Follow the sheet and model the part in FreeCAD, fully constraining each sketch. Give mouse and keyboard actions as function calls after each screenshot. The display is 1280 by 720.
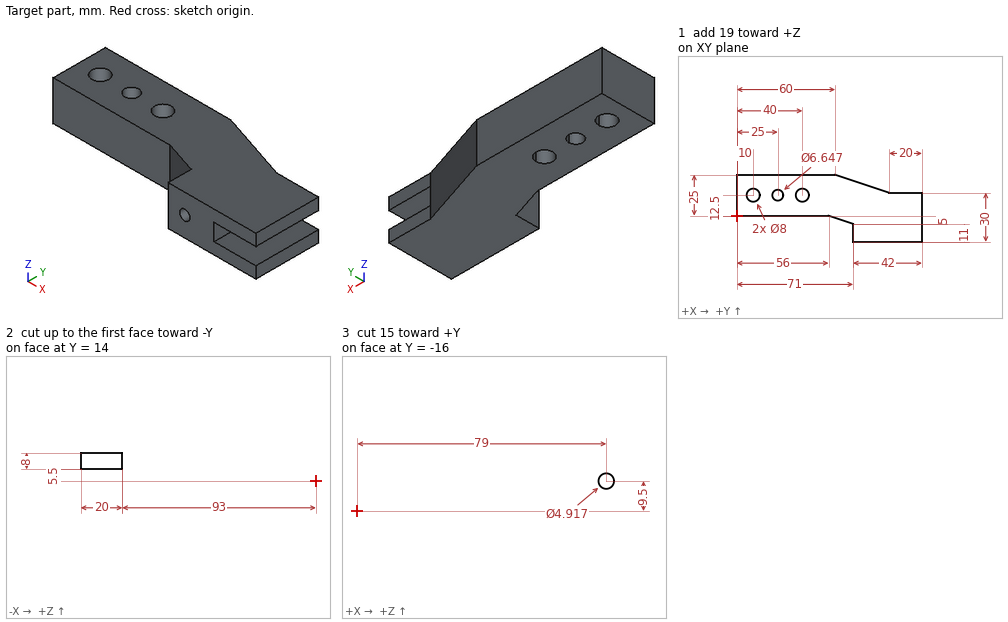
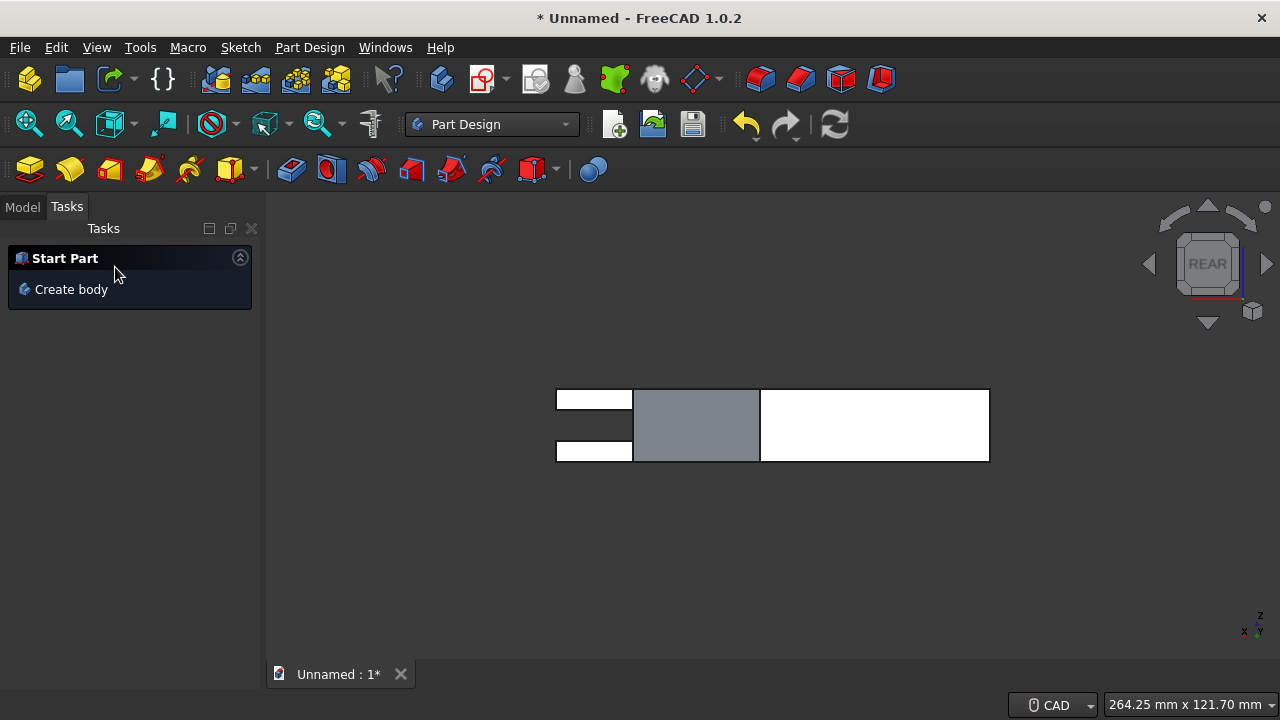
key(0)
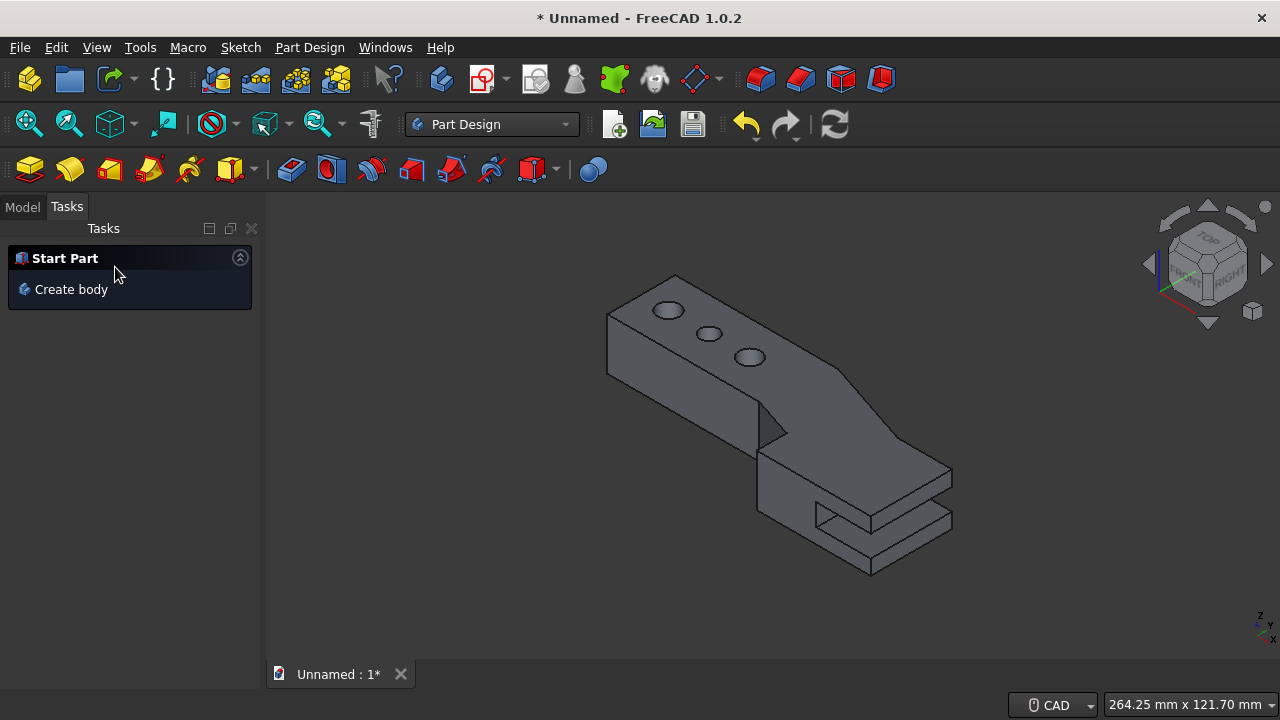
click(781, 493)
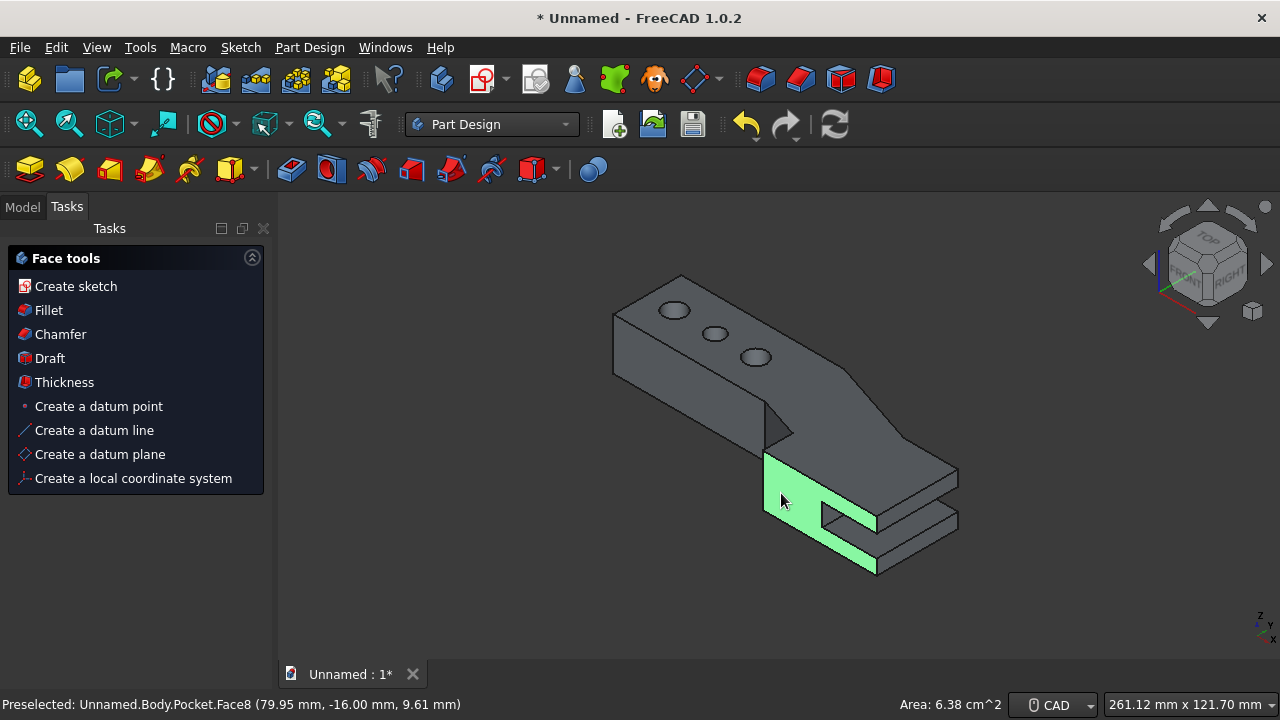
click(482, 80)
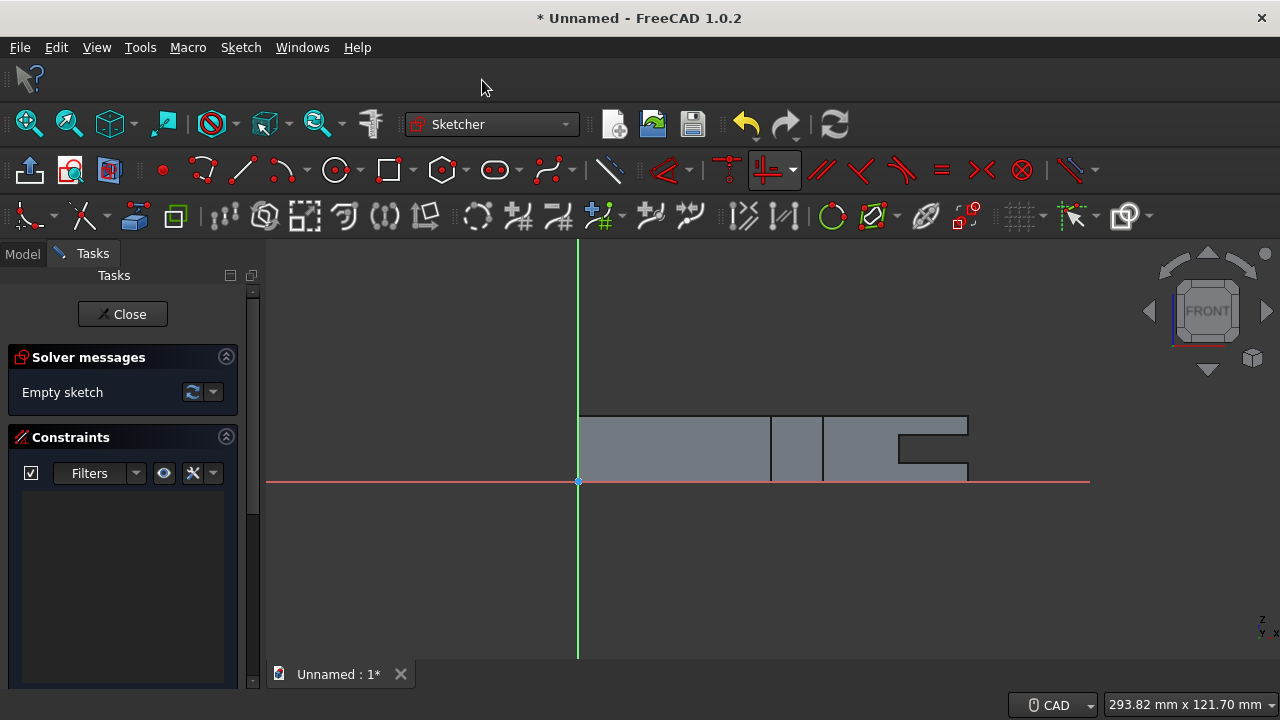
scroll(860, 449, up, 14)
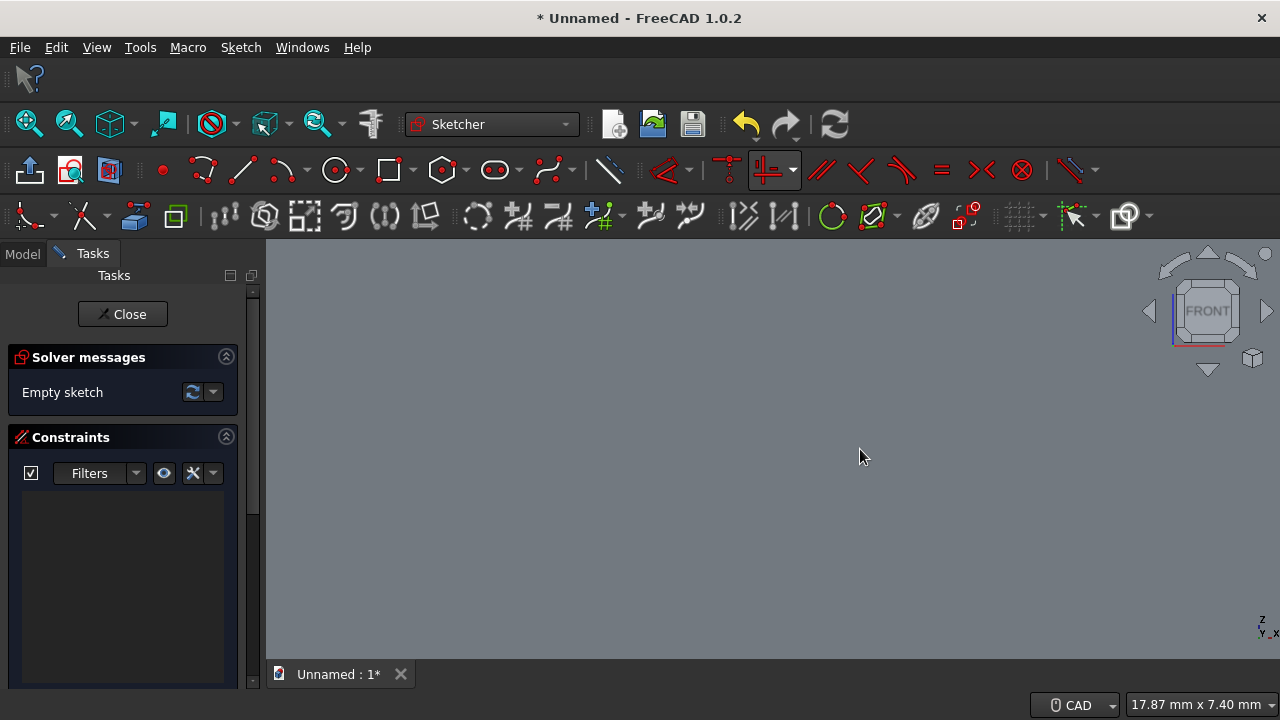
click(336, 170)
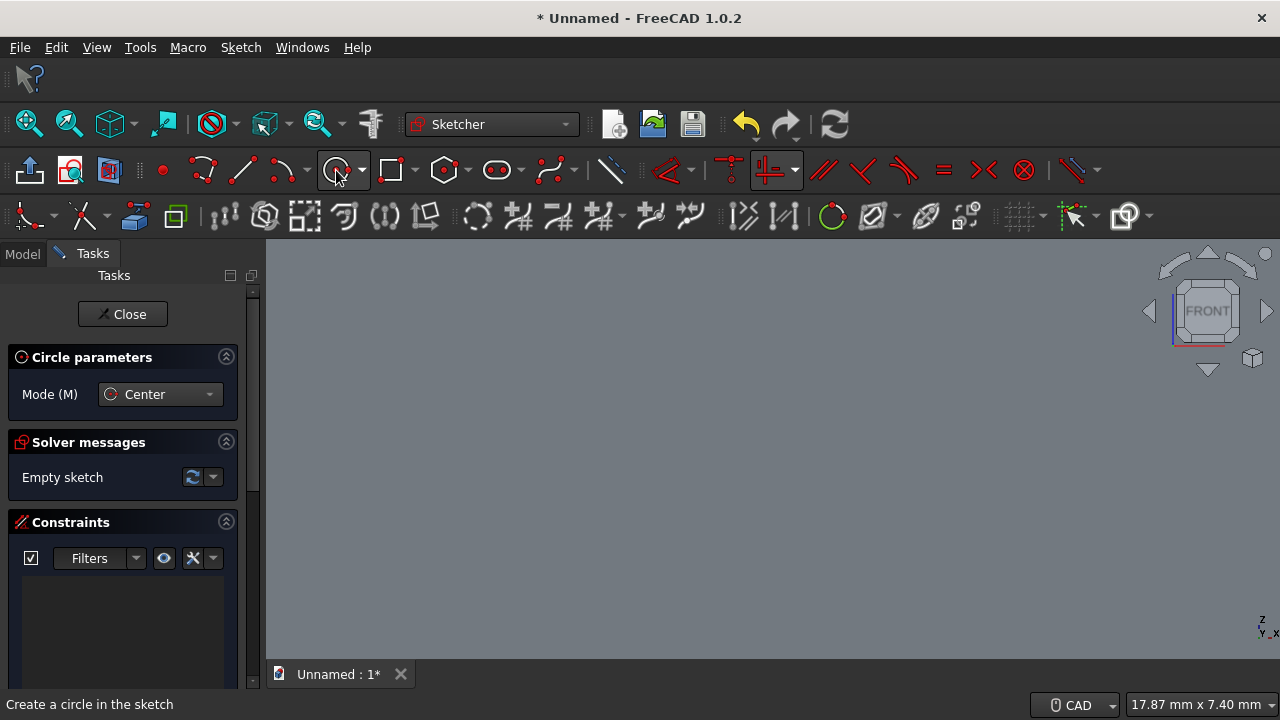
click(697, 441)
click(796, 343)
key(Escape)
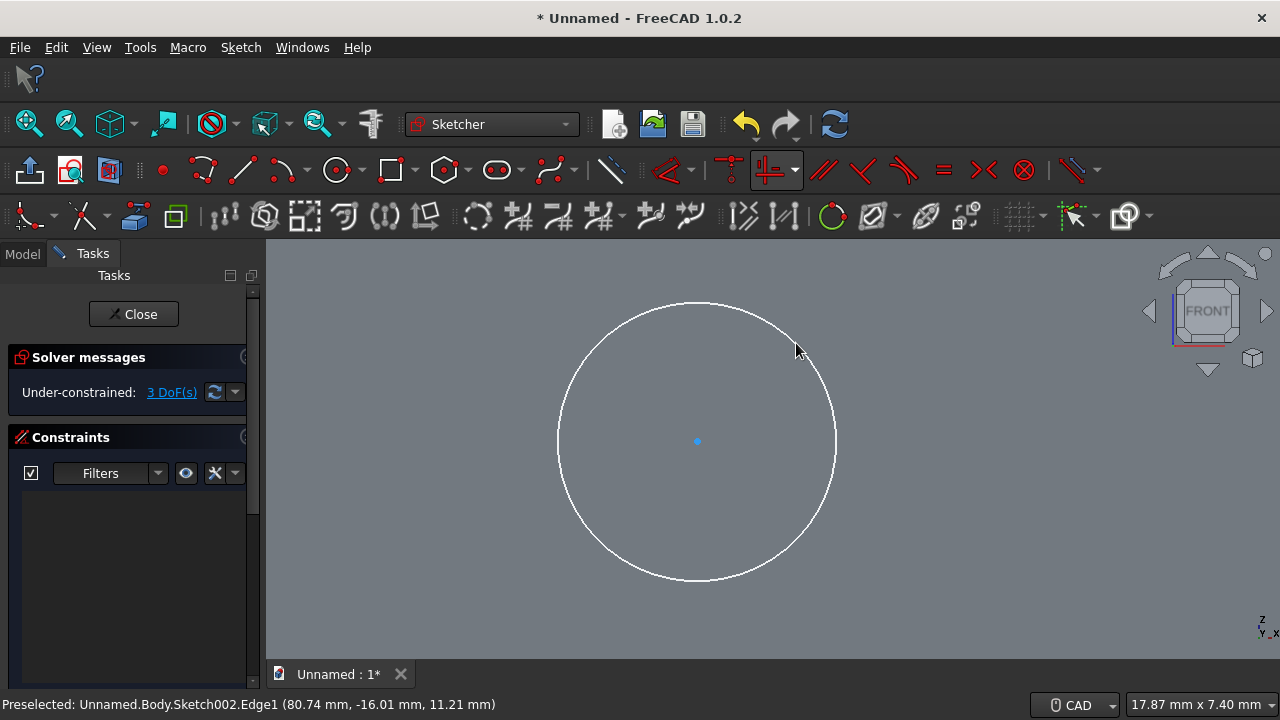
click(666, 170)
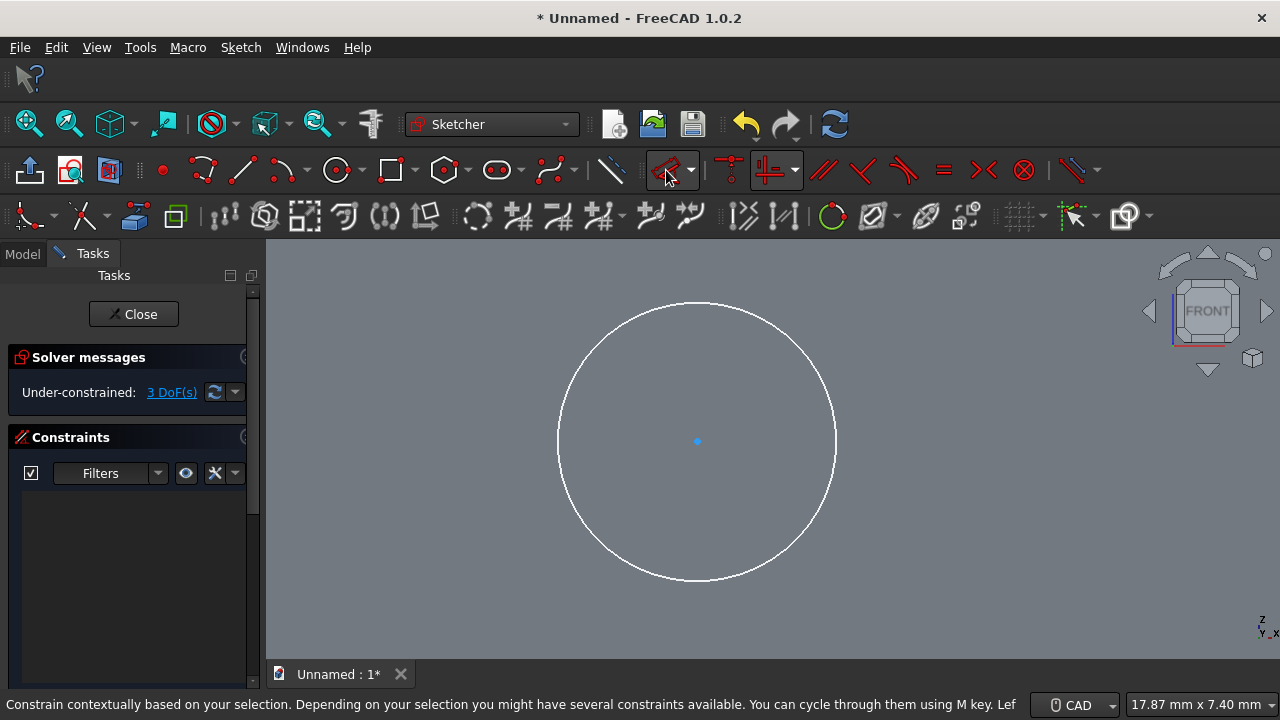
click(795, 343)
click(818, 320)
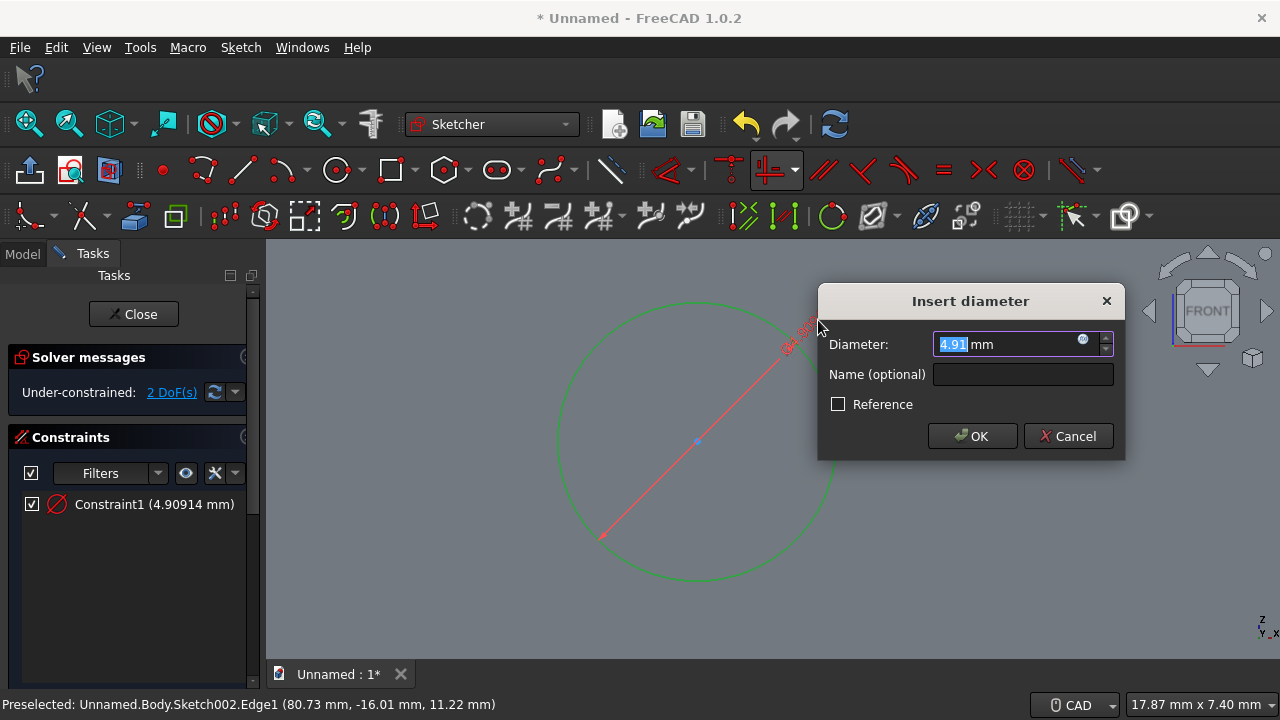
text(4.917)
key(Return)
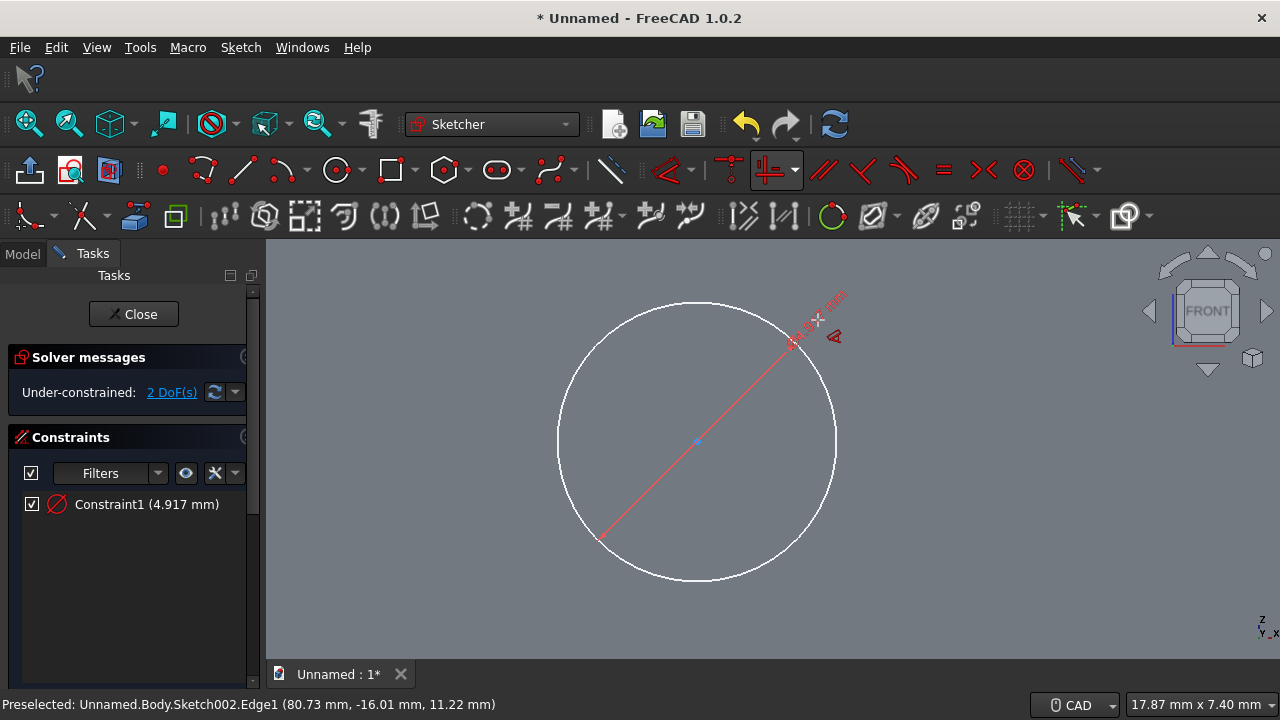
click(697, 442)
click(496, 408)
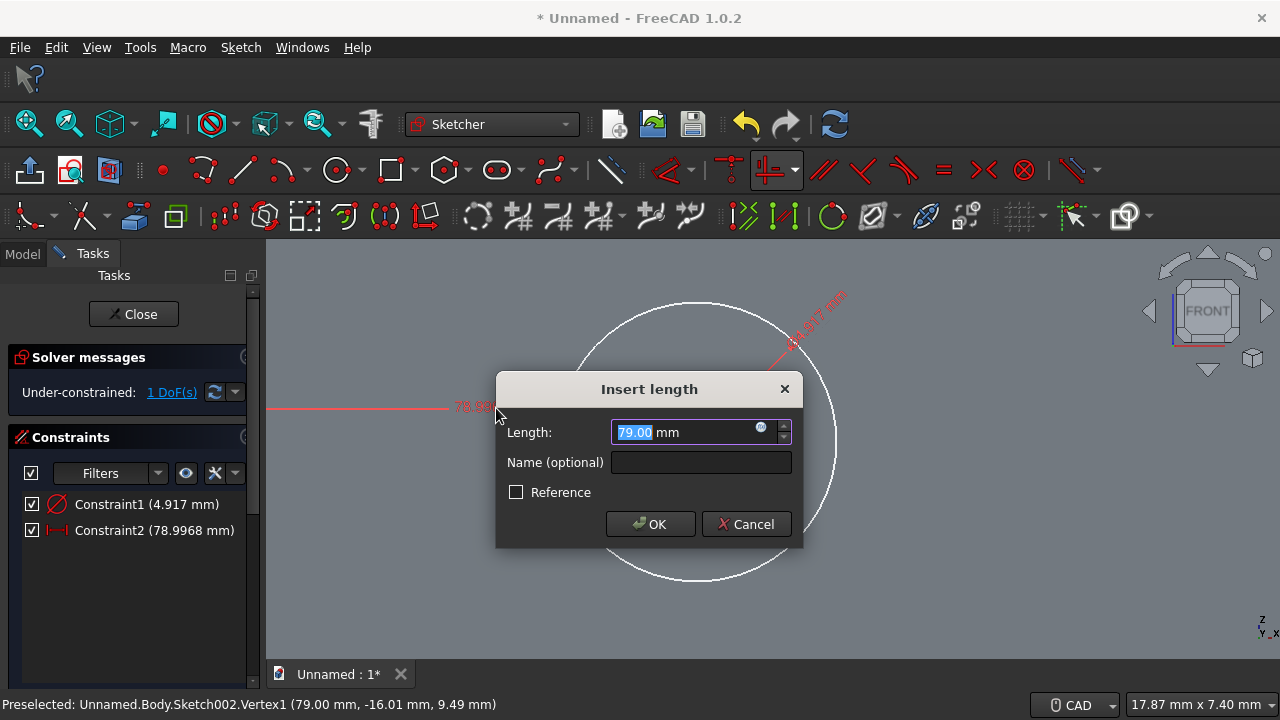
text(79)
key(Return)